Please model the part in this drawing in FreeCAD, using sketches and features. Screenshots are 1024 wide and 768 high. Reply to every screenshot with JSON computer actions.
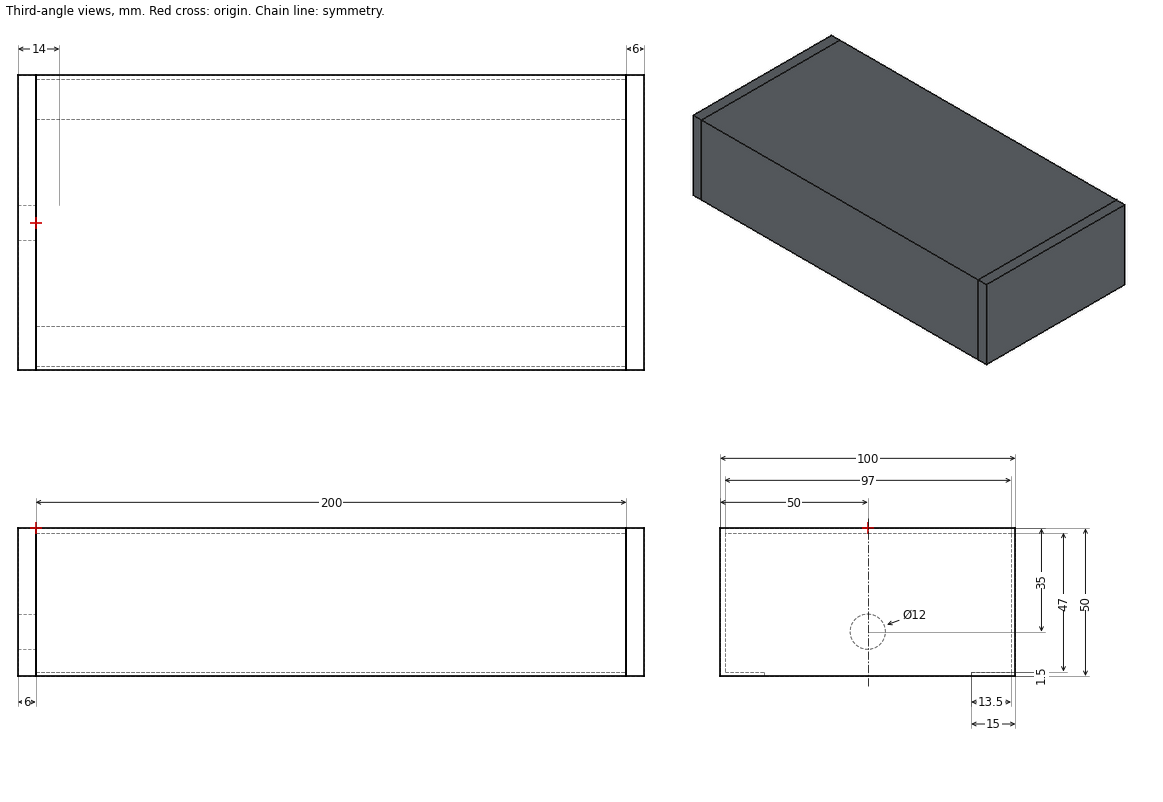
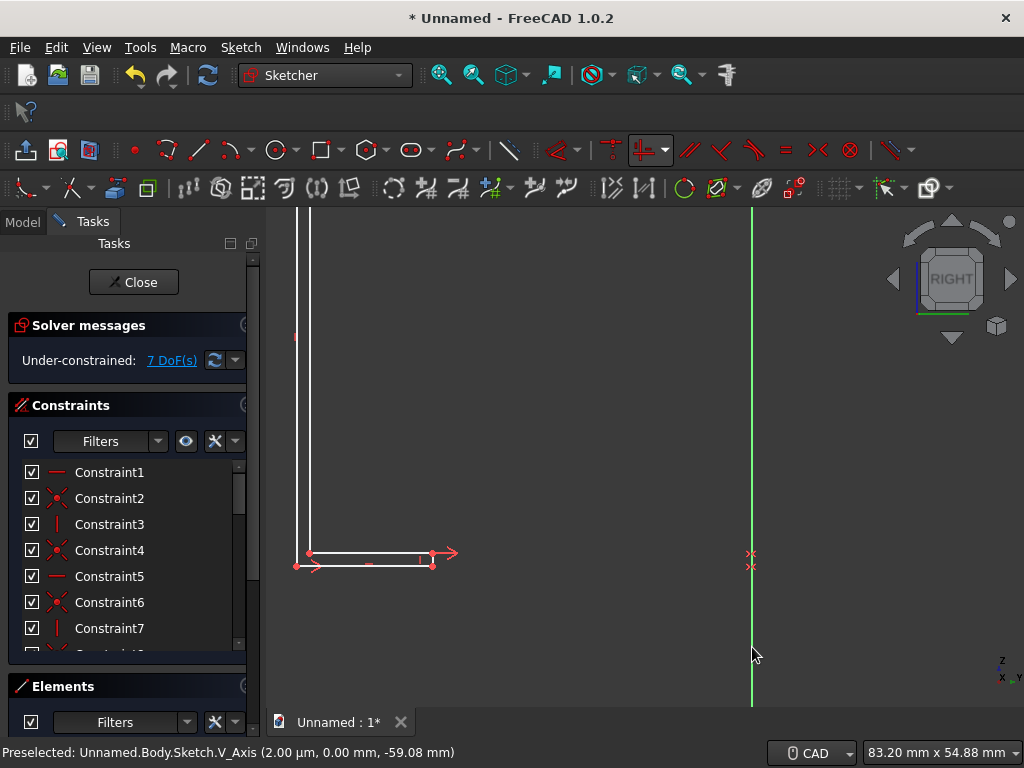
{"action": "left_click", "coordinate": [556, 150]}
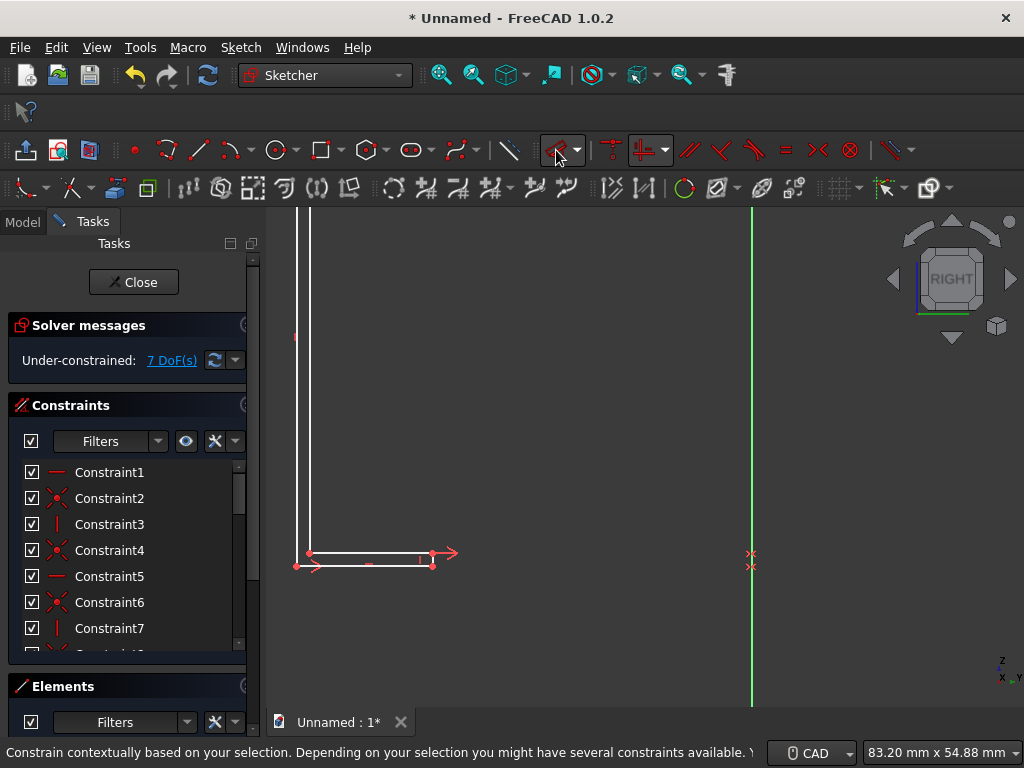
{"action": "scroll", "coordinate": [433, 554], "scroll_direction": "down", "scroll_amount": 4}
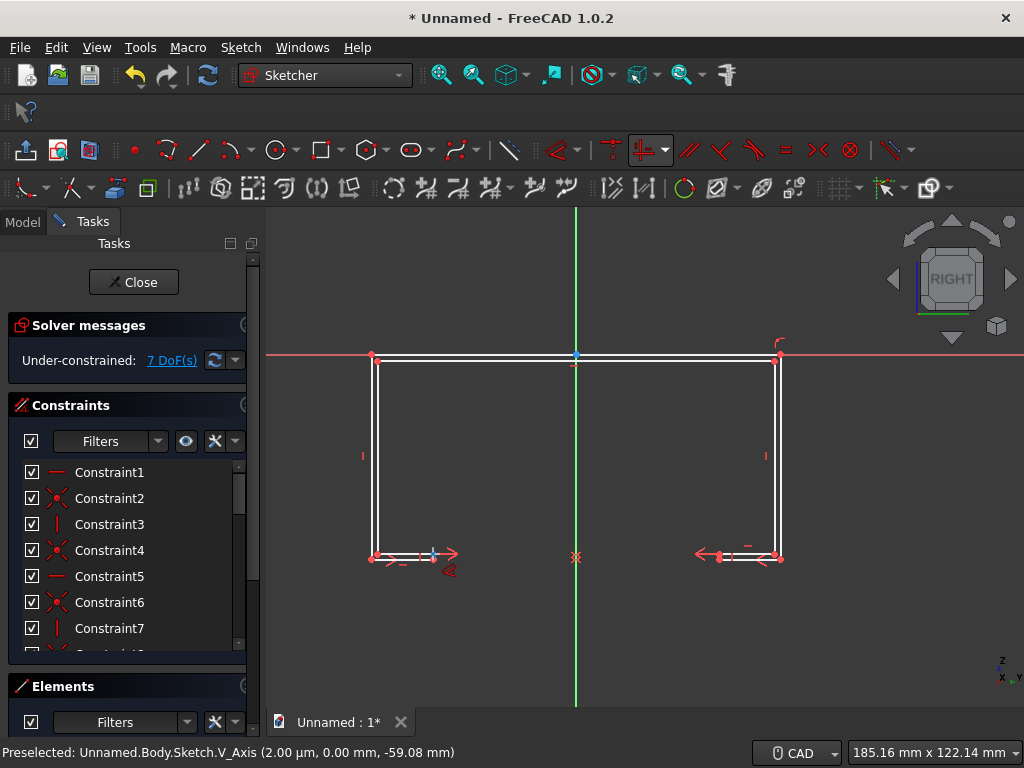
{"action": "scroll", "coordinate": [497, 361], "scroll_direction": "up", "scroll_amount": 4}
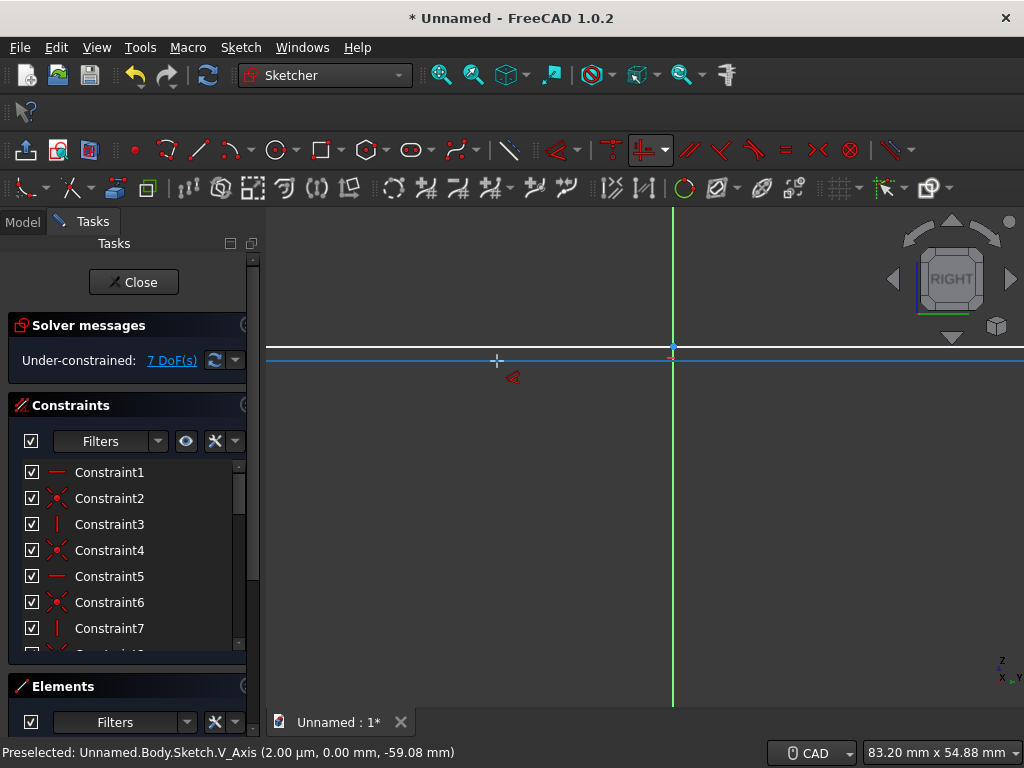
{"action": "left_click", "coordinate": [496, 361]}
{"action": "left_click", "coordinate": [576, 327]}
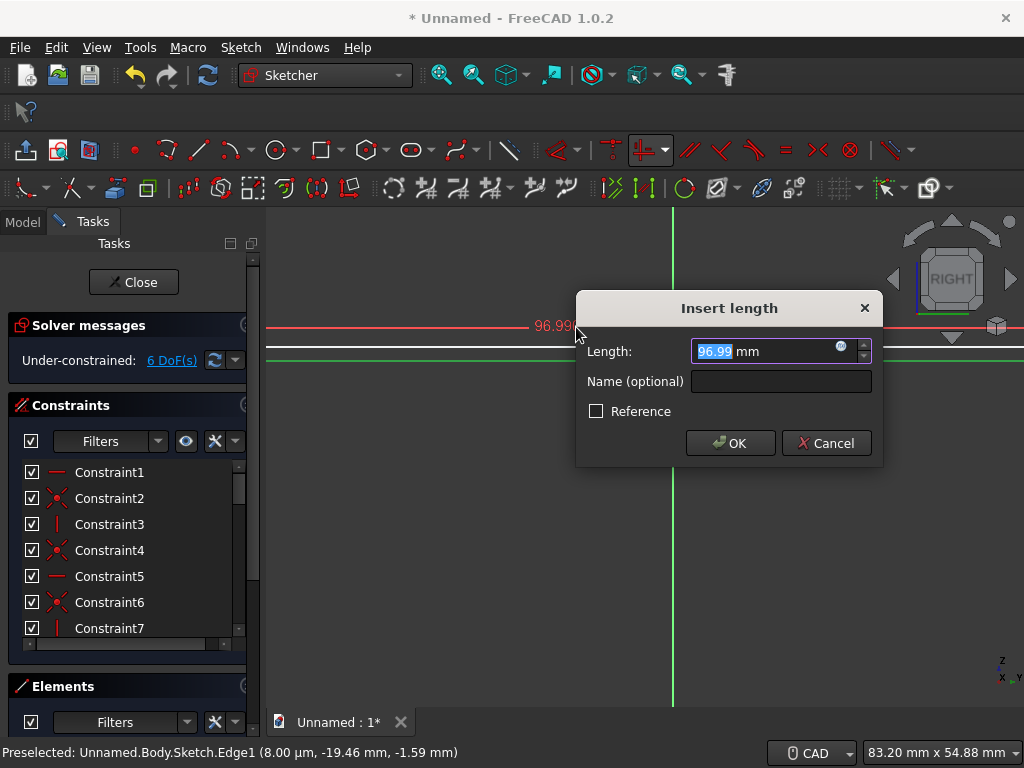
{"action": "type", "text": "97"}
{"action": "key", "text": "Return"}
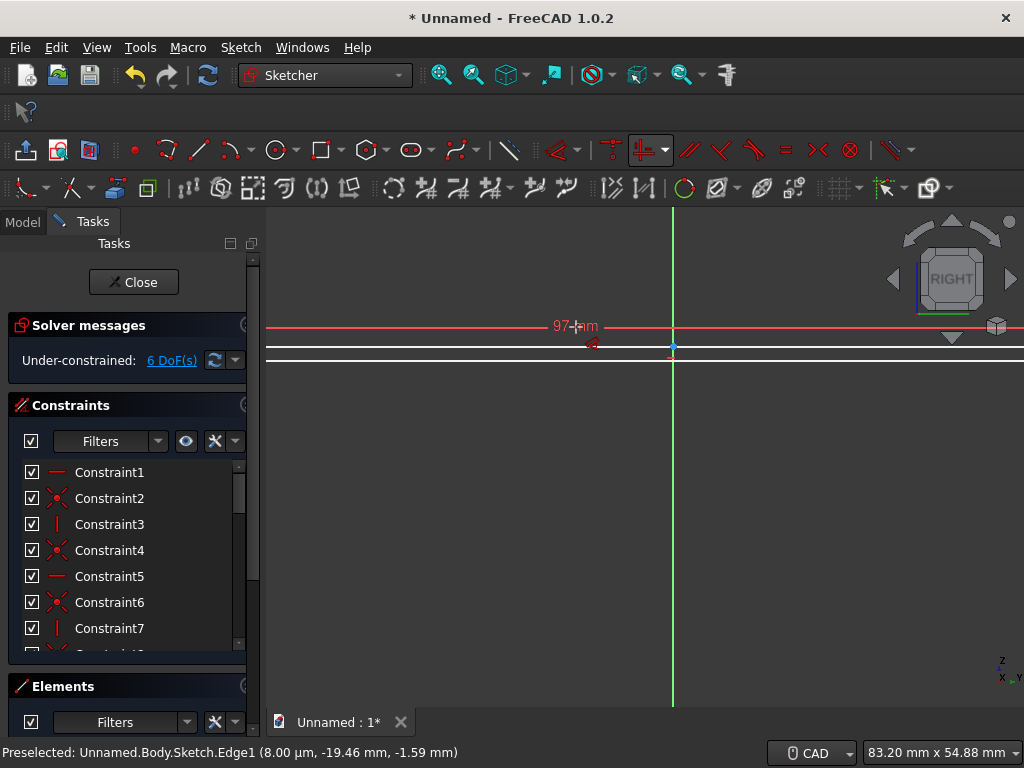
{"action": "scroll", "coordinate": [497, 361], "scroll_direction": "down", "scroll_amount": 4}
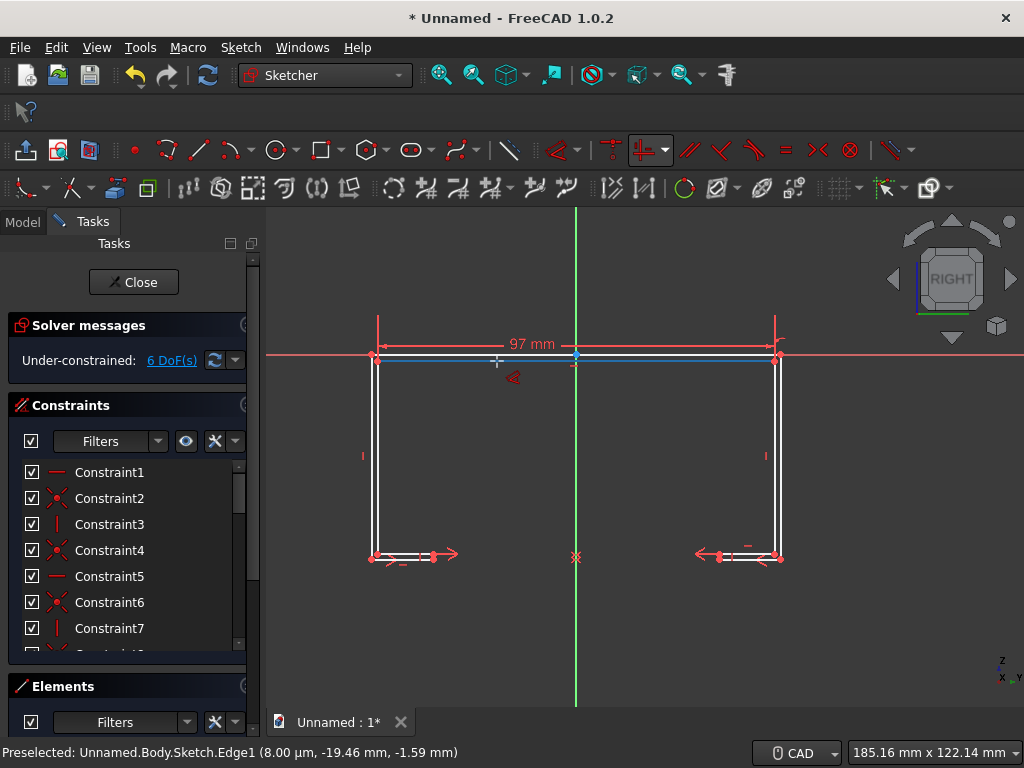
{"action": "scroll", "coordinate": [775, 419], "scroll_direction": "up", "scroll_amount": 5}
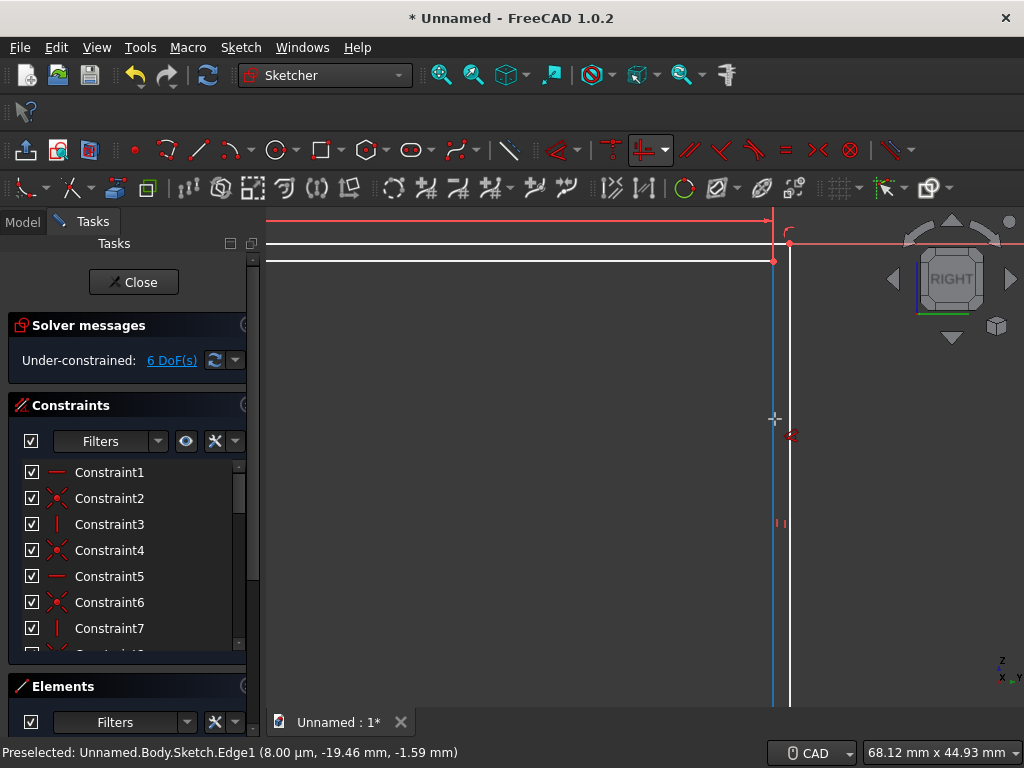
{"action": "left_click", "coordinate": [773, 419]}
{"action": "left_click", "coordinate": [807, 470]}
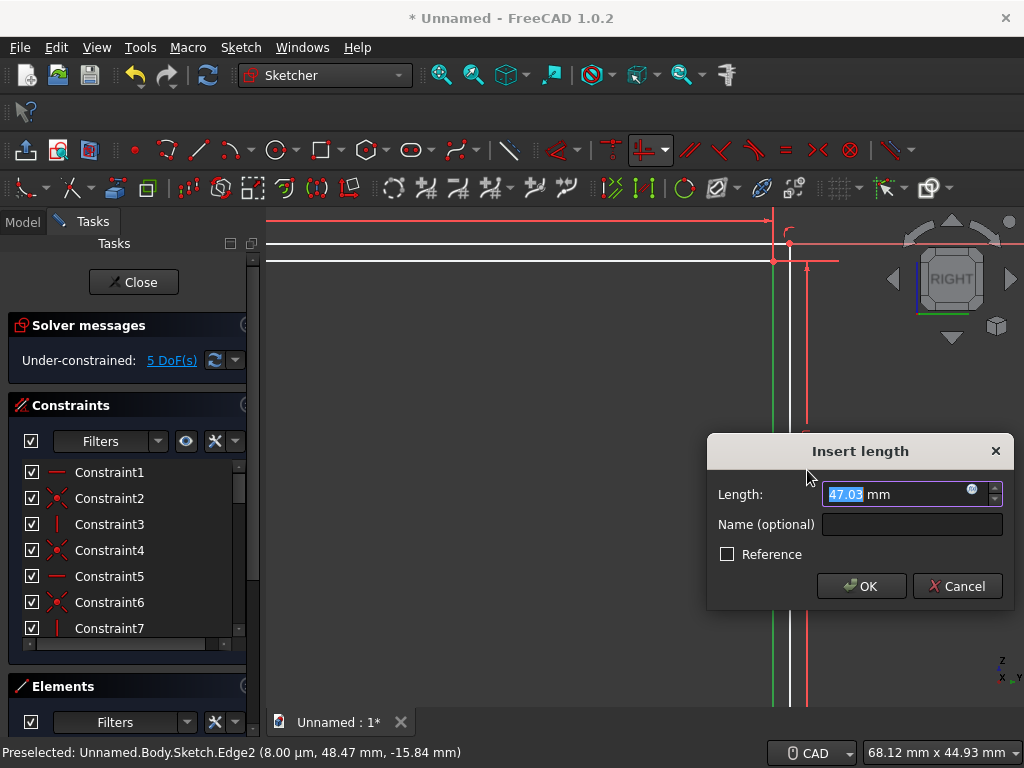
{"action": "type", "text": "47"}
{"action": "key", "text": "Return"}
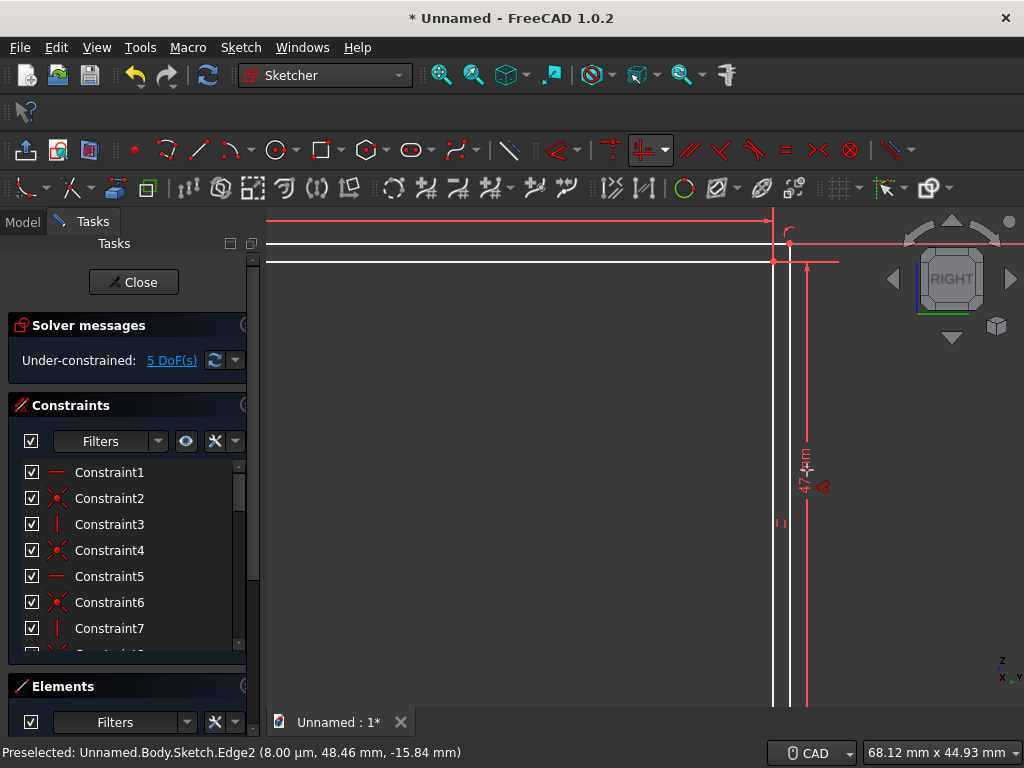
{"action": "scroll", "coordinate": [776, 419], "scroll_direction": "down", "scroll_amount": 5}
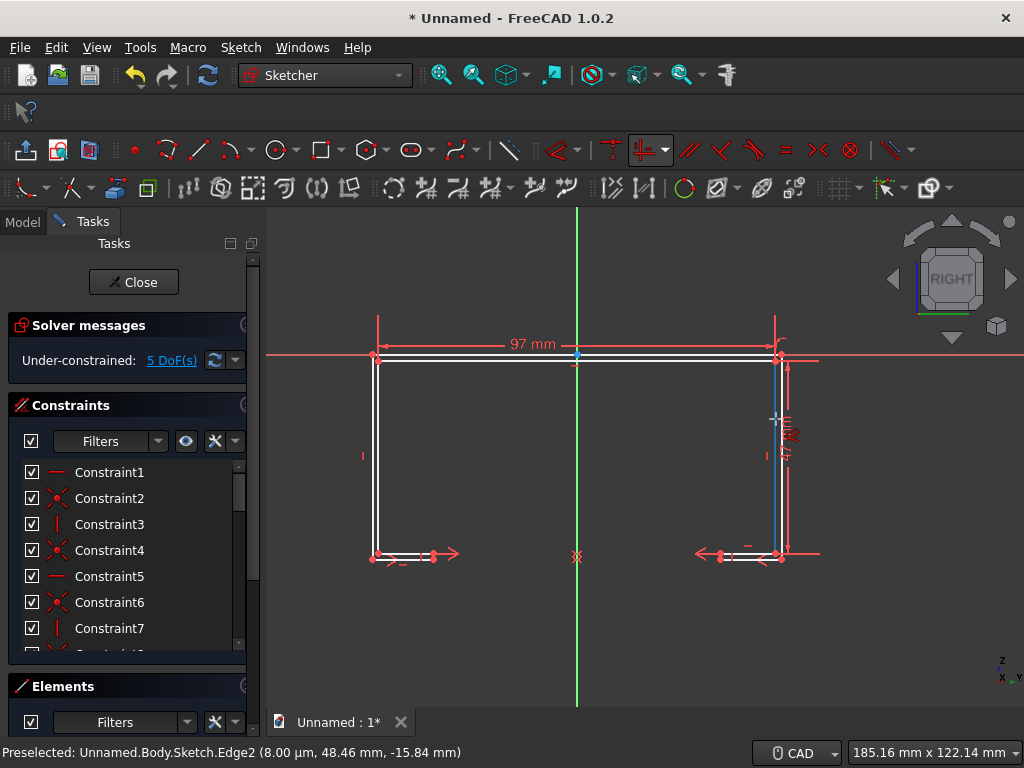
{"action": "scroll", "coordinate": [739, 560], "scroll_direction": "up", "scroll_amount": 5}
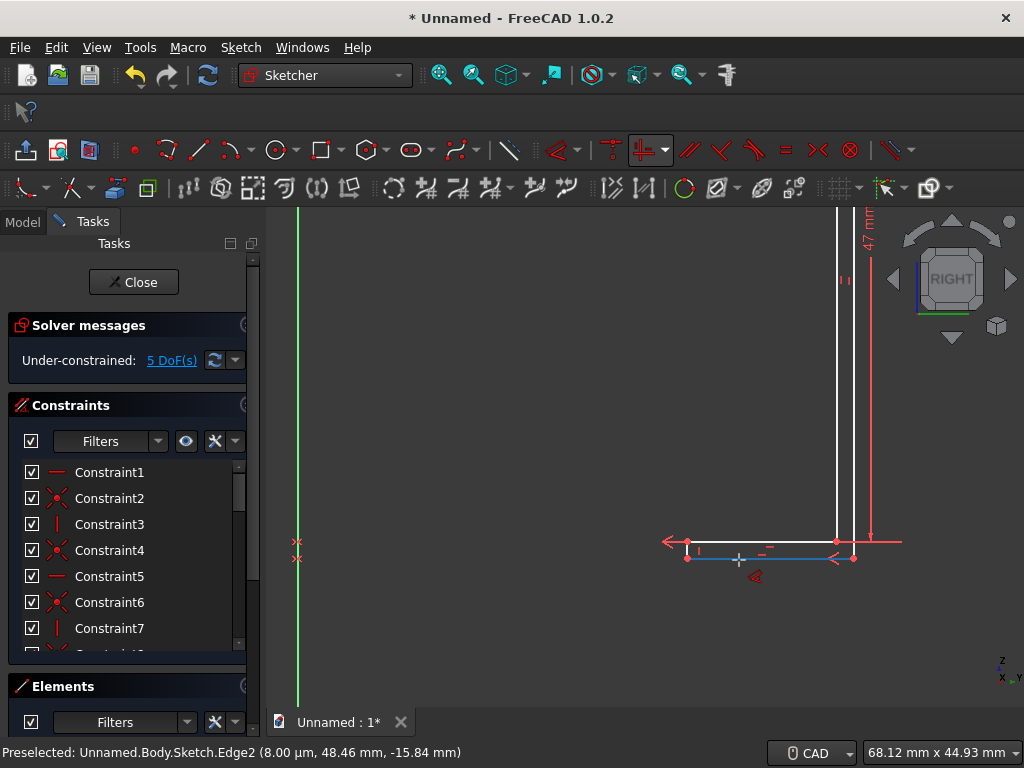
{"action": "left_click", "coordinate": [737, 559]}
{"action": "left_click", "coordinate": [771, 593]}